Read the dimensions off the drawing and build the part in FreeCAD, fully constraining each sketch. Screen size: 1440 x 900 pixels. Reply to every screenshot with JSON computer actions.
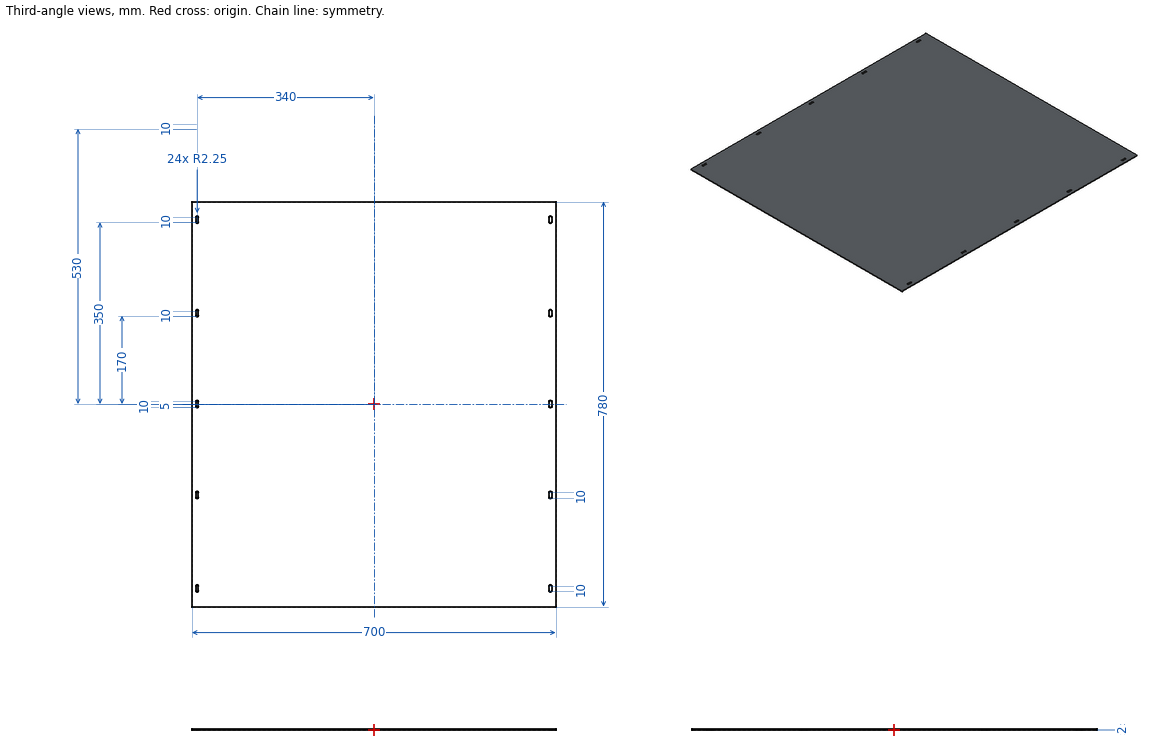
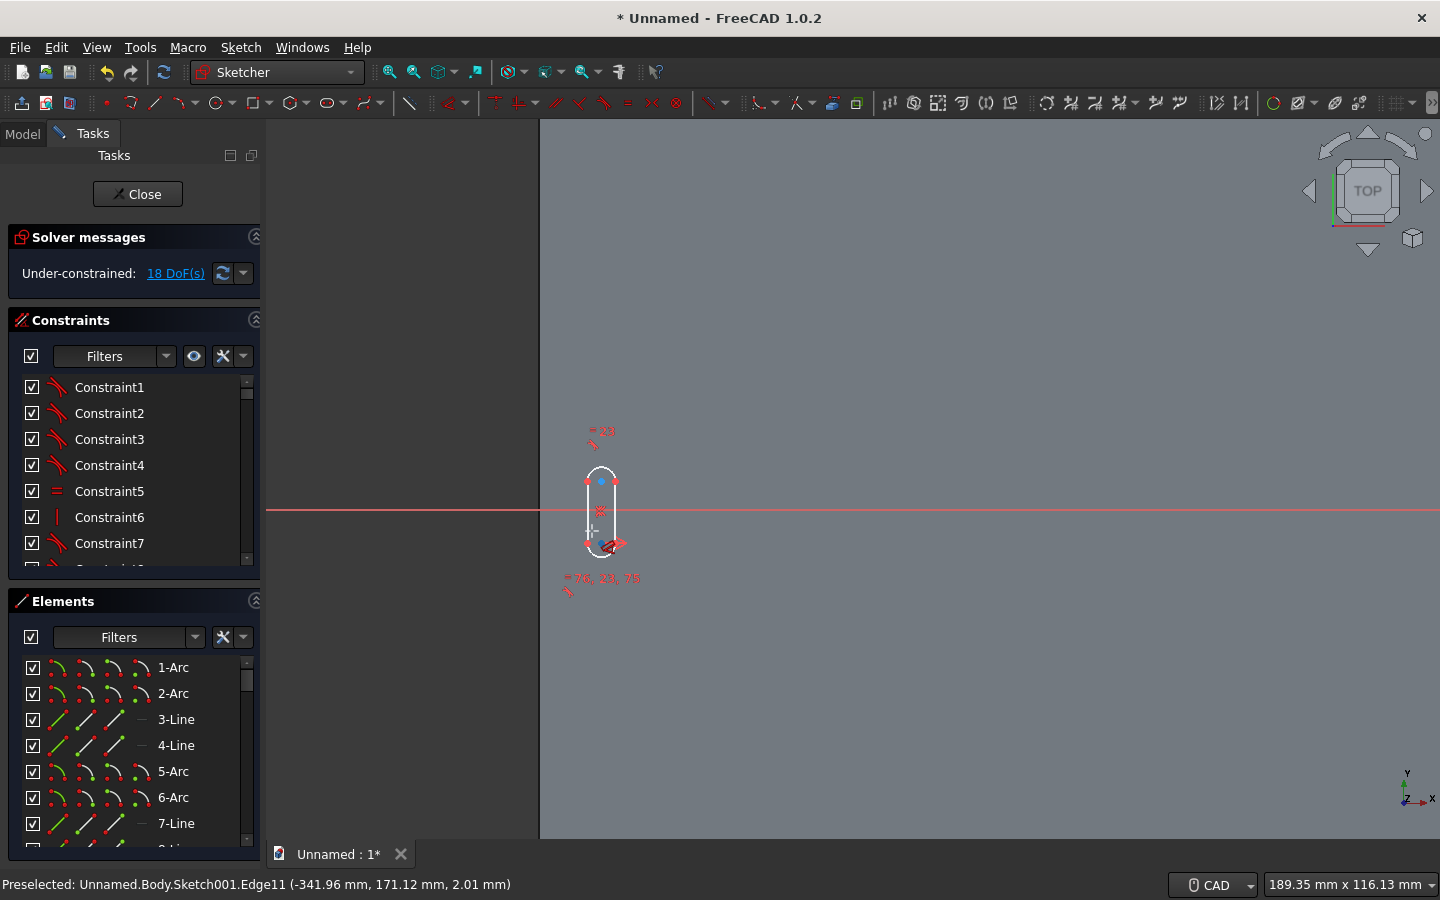
{"action": "left_click", "coordinate": [588, 525]}
{"action": "left_click", "coordinate": [554, 526]}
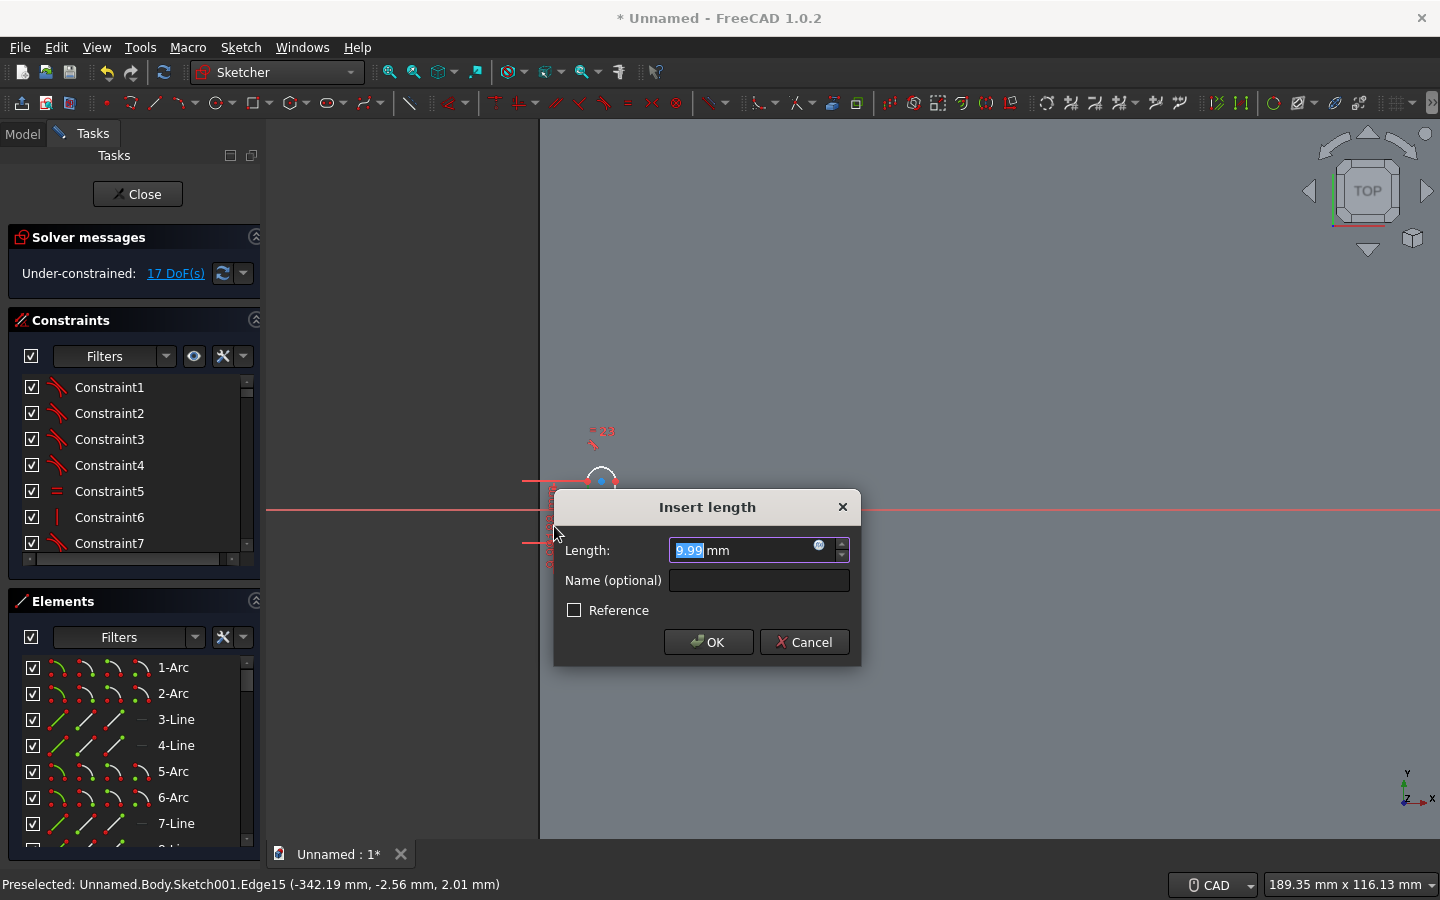
{"action": "type", "text": "10"}
{"action": "key", "text": "Return"}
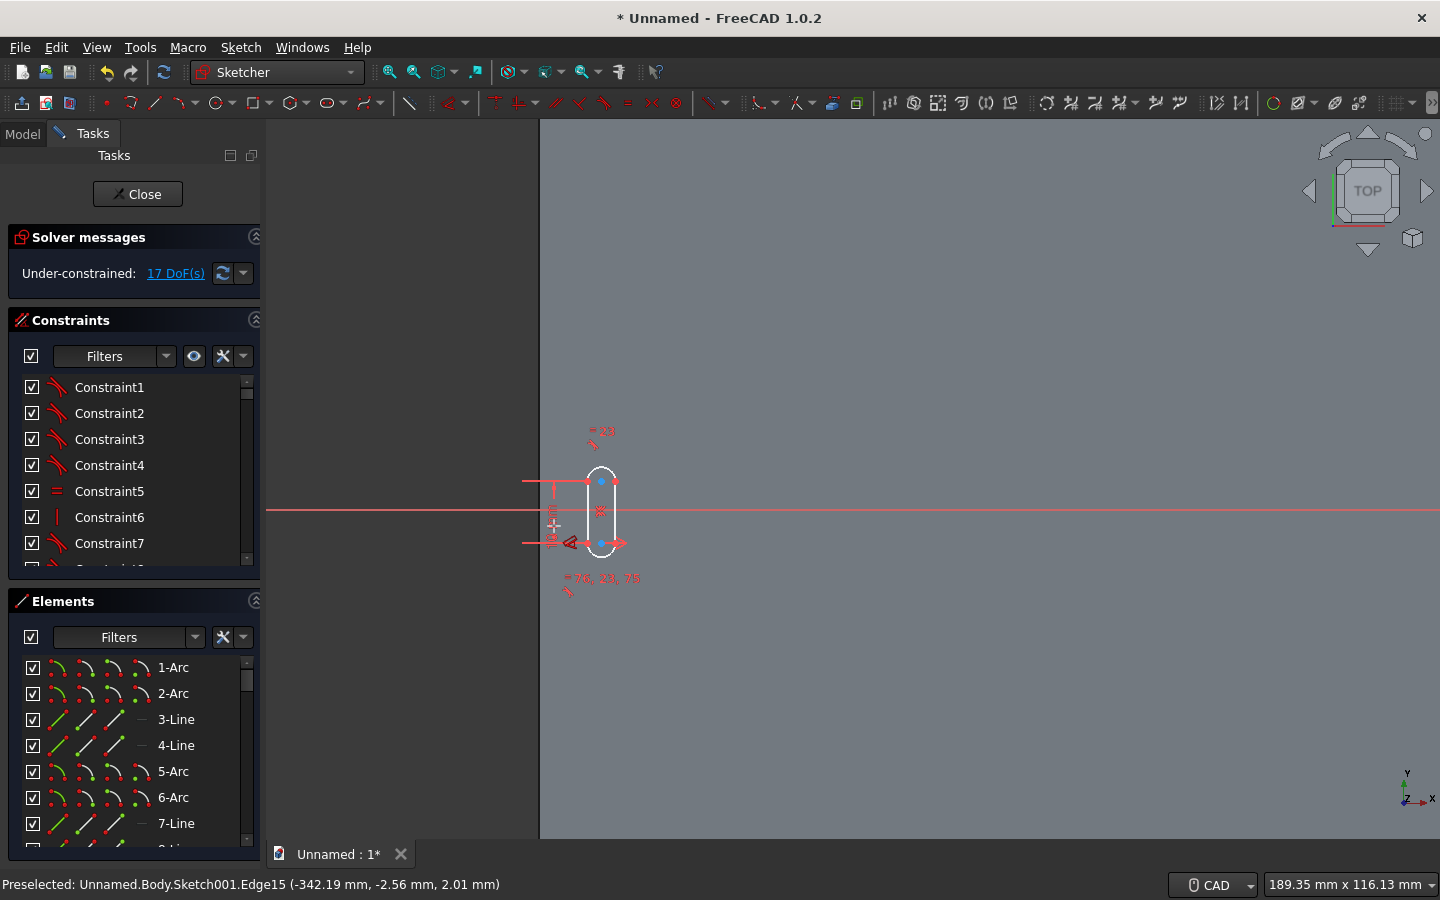
{"action": "scroll", "coordinate": [592, 532], "scroll_direction": "down", "scroll_amount": 12}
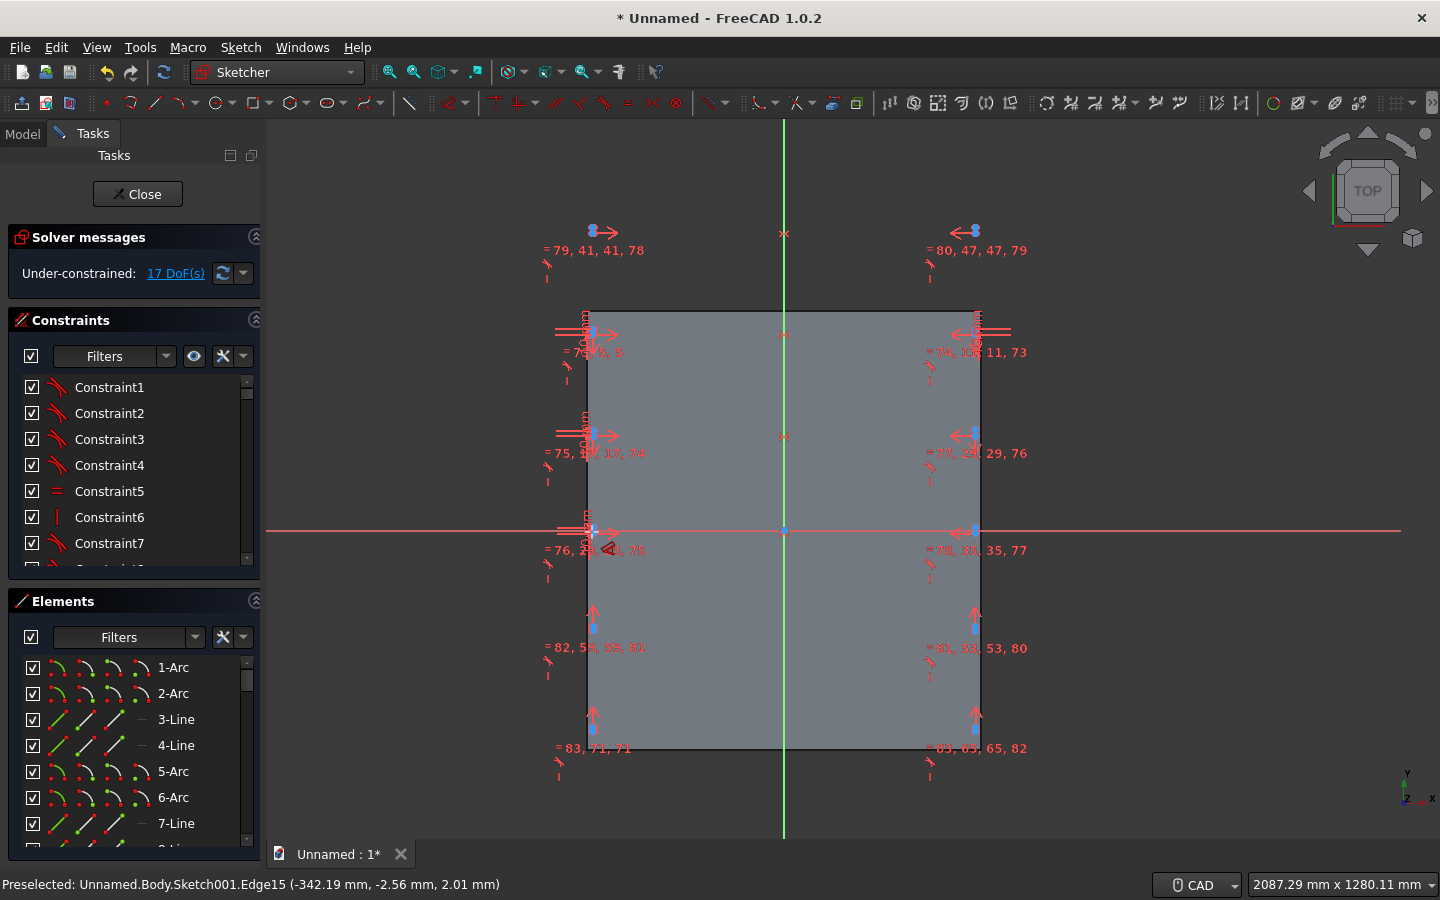
{"action": "scroll", "coordinate": [974, 434], "scroll_direction": "up", "scroll_amount": 10}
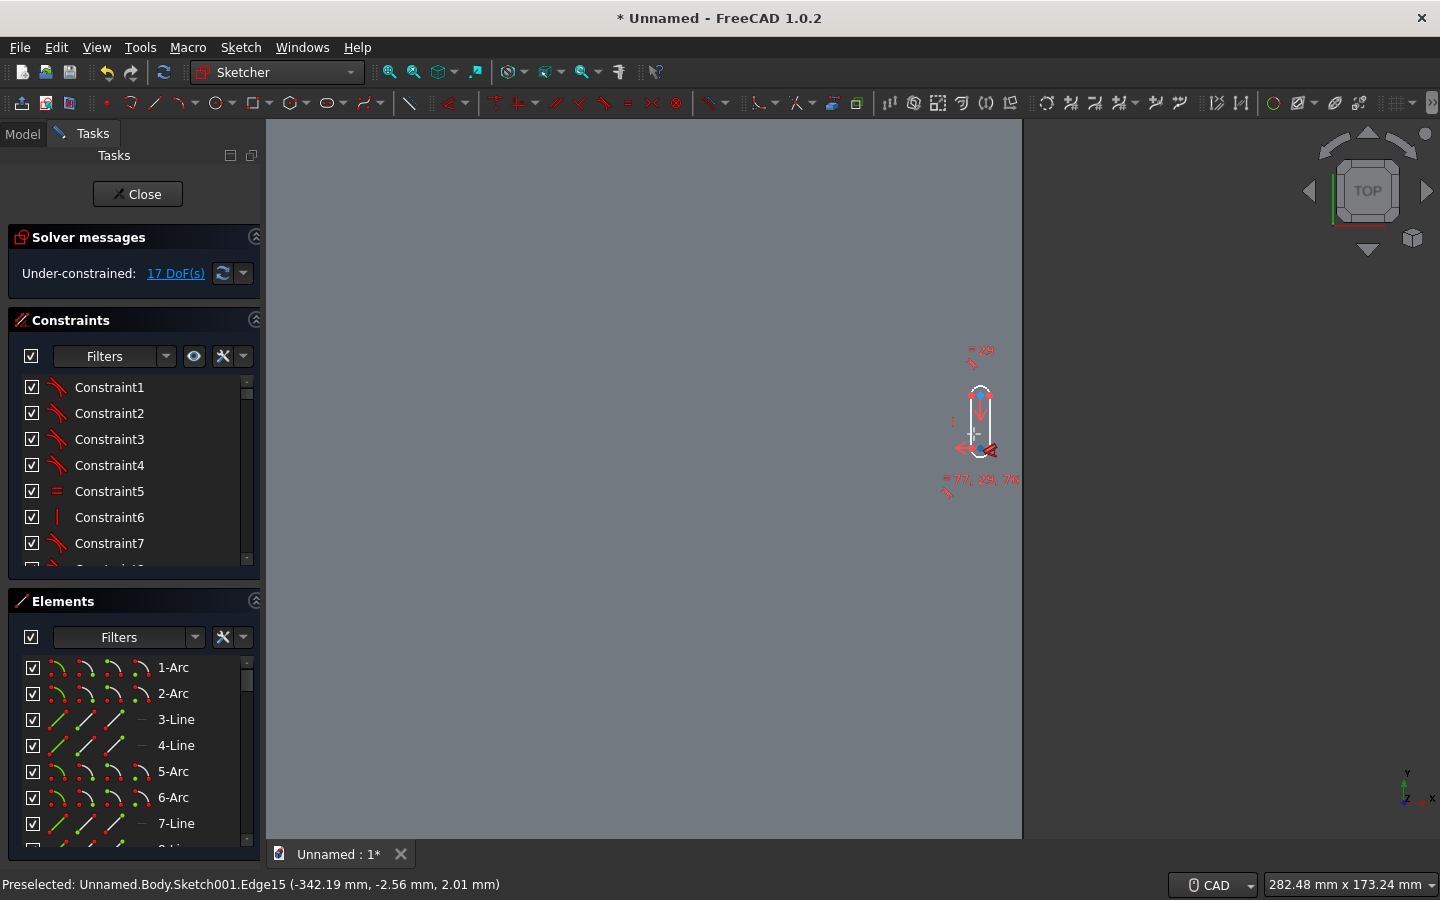
{"action": "left_click", "coordinate": [971, 432]}
{"action": "left_click", "coordinate": [1005, 422]}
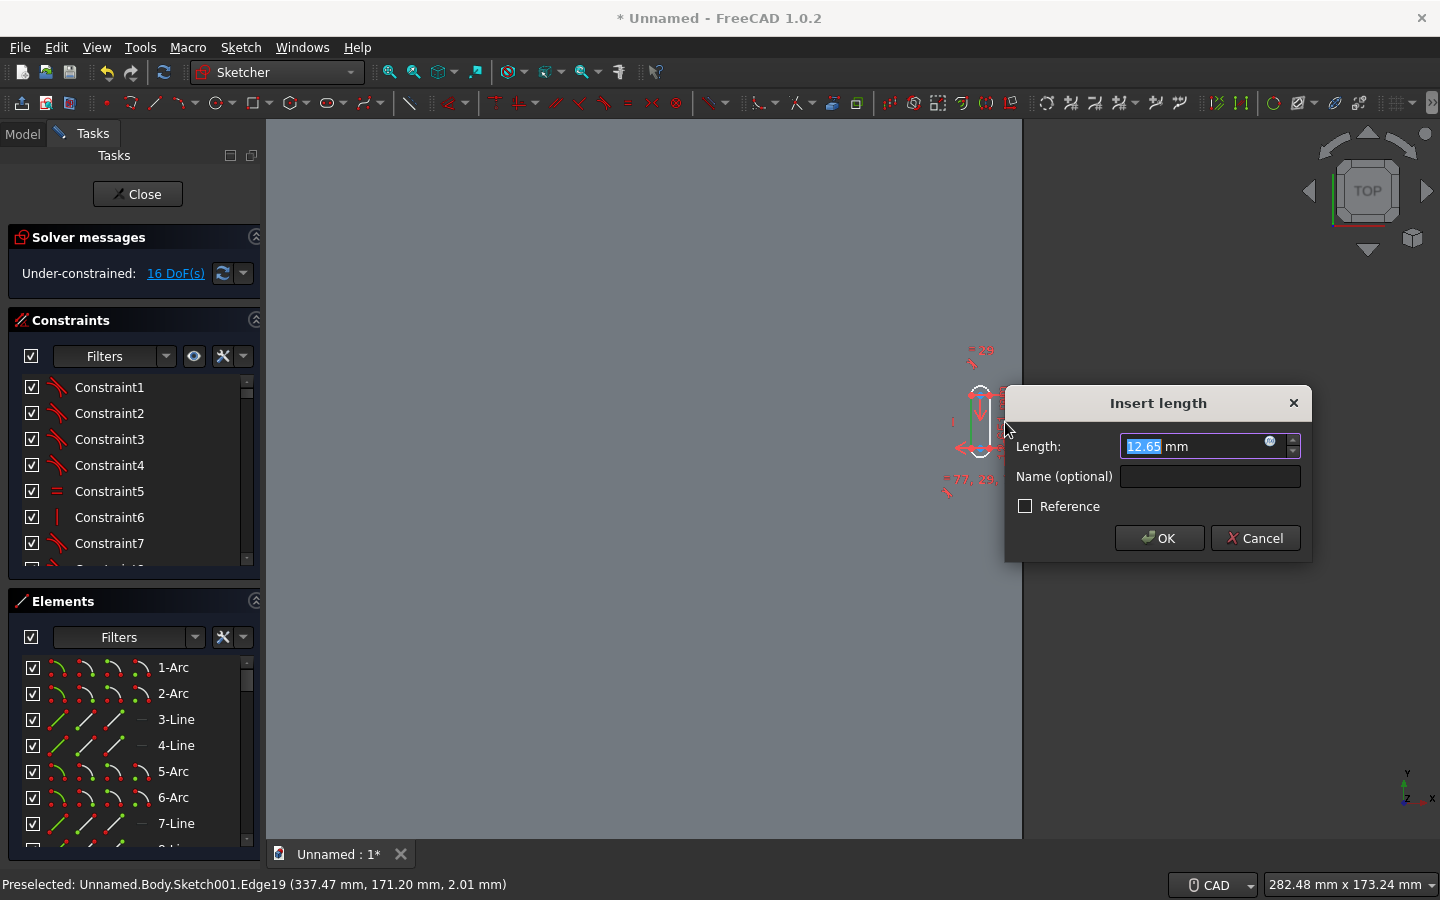
{"action": "type", "text": "10"}
{"action": "key", "text": "Return"}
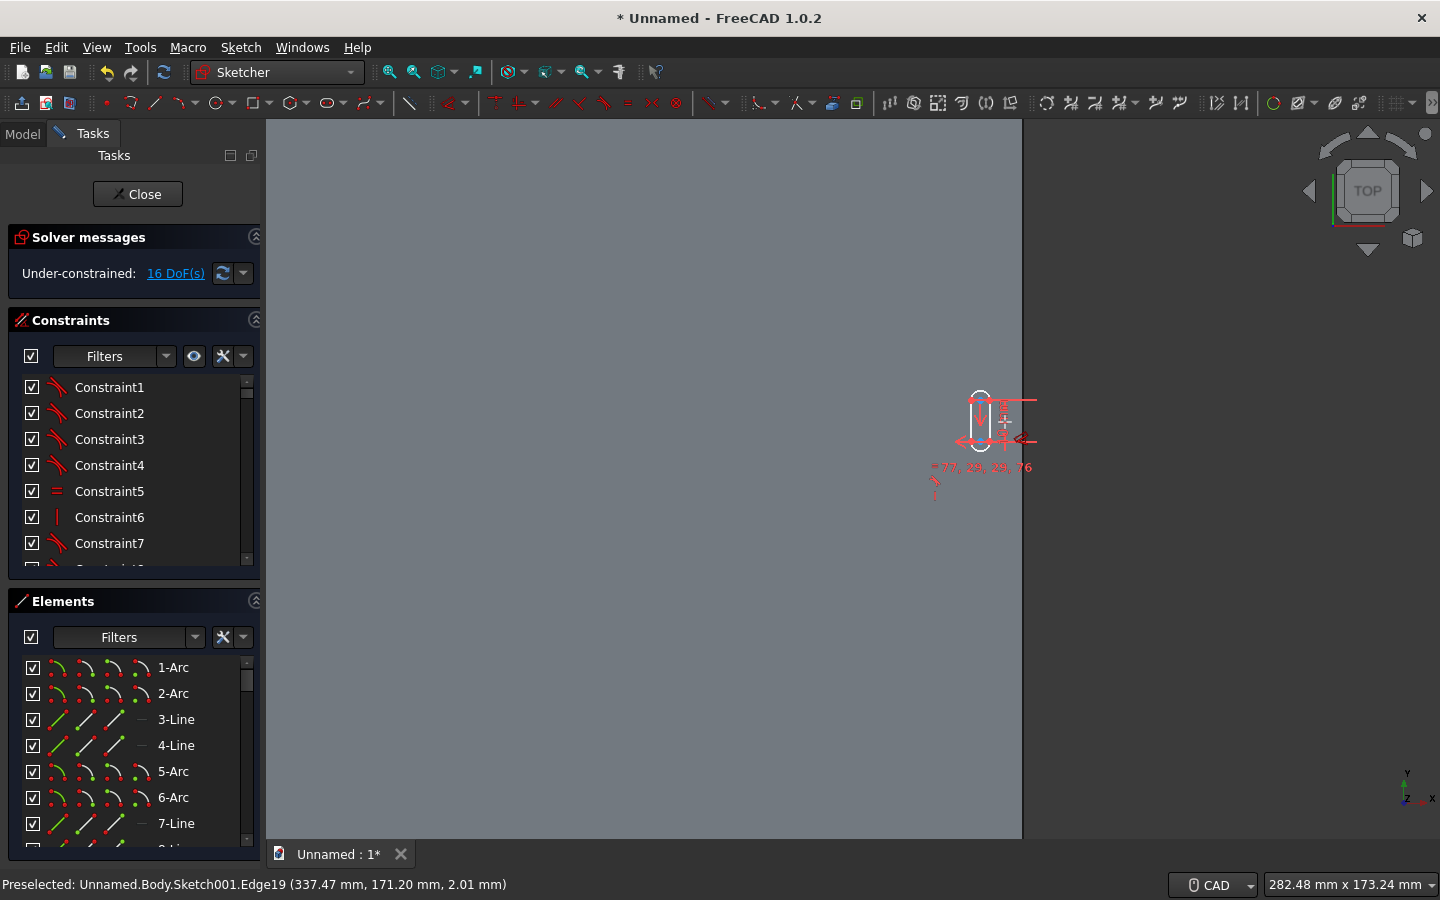
{"action": "scroll", "coordinate": [975, 433], "scroll_direction": "down", "scroll_amount": 10}